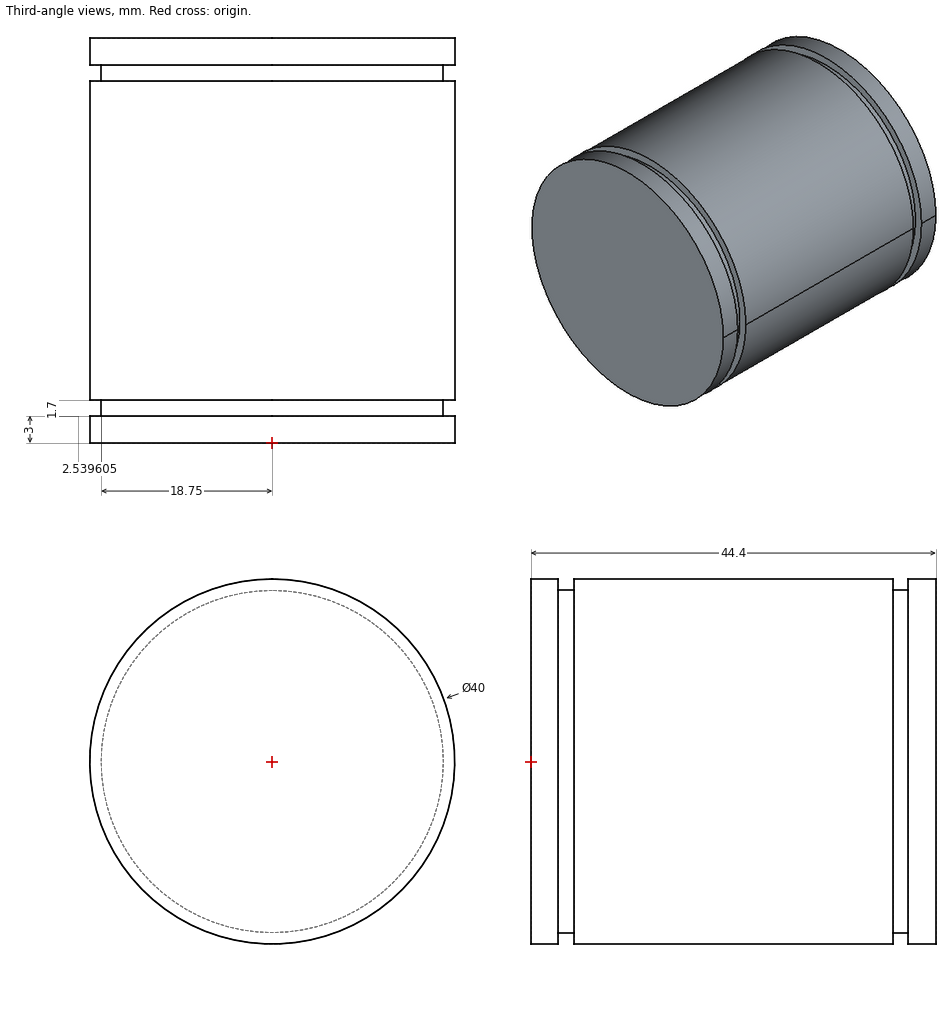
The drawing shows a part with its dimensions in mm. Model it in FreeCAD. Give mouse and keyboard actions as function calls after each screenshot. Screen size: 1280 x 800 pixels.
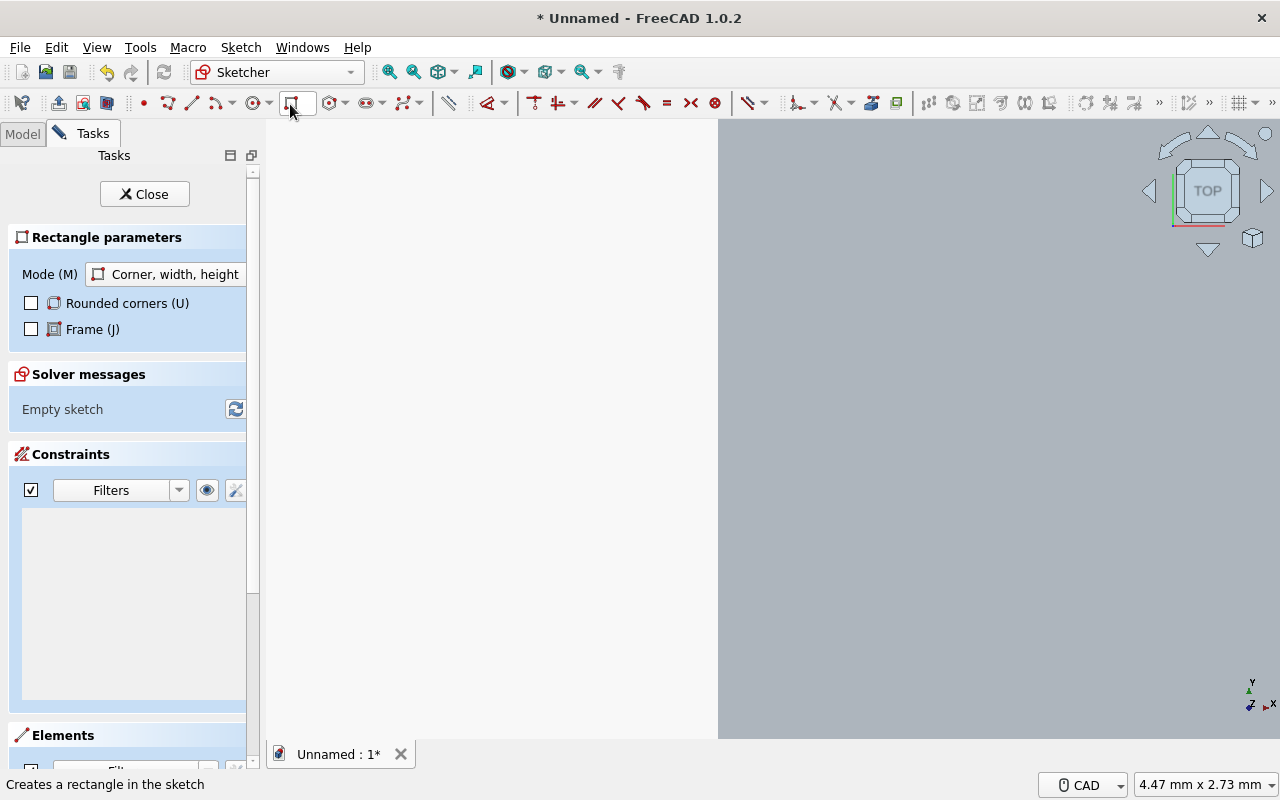
click(416, 236)
move(992, 622)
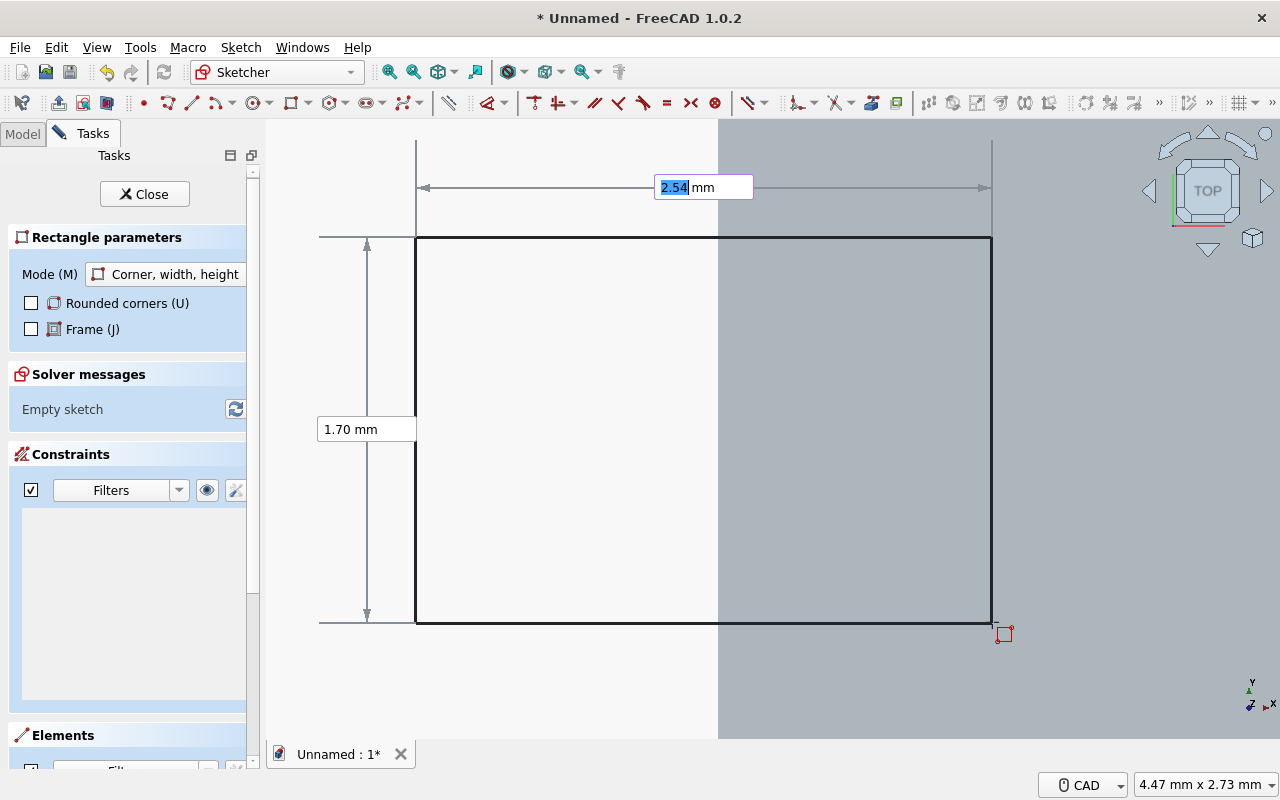
text(2.539605)
key(Tab)
text(1.7)
key(Return)
key(Escape)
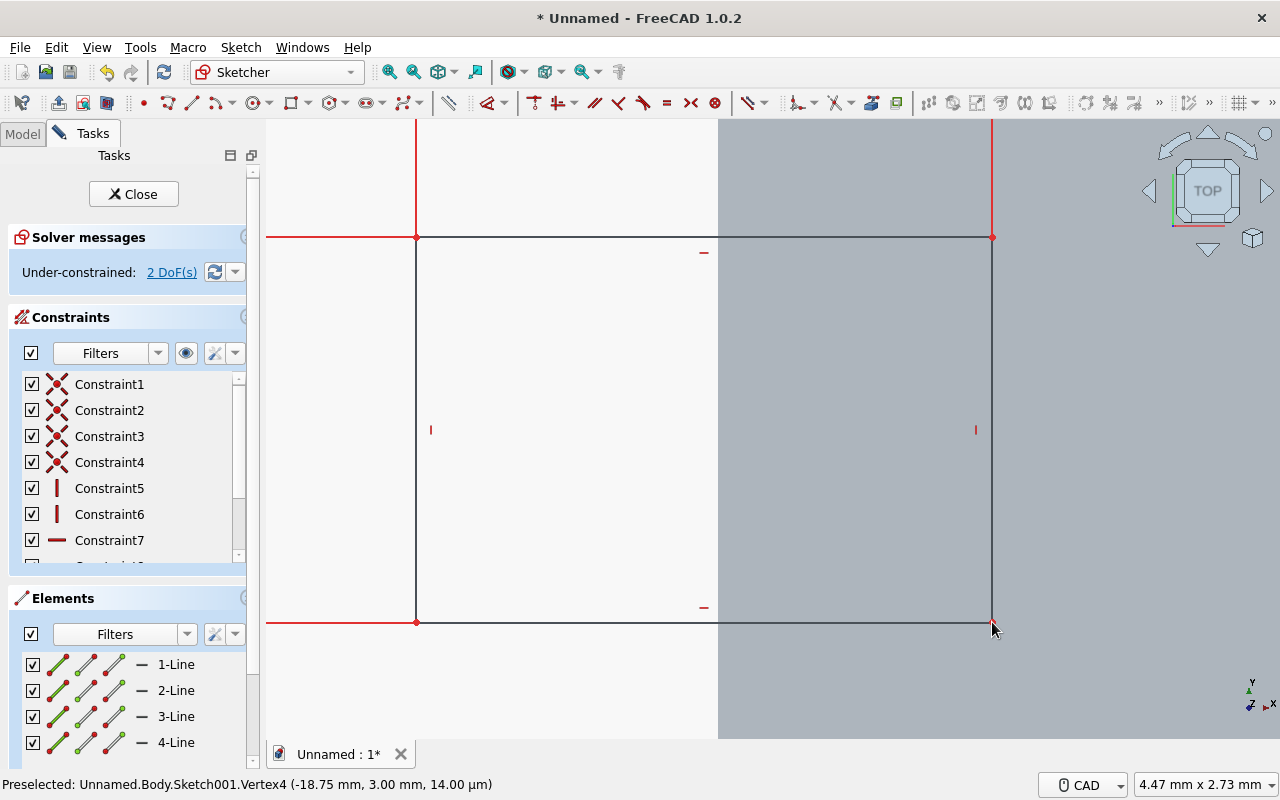
key(d)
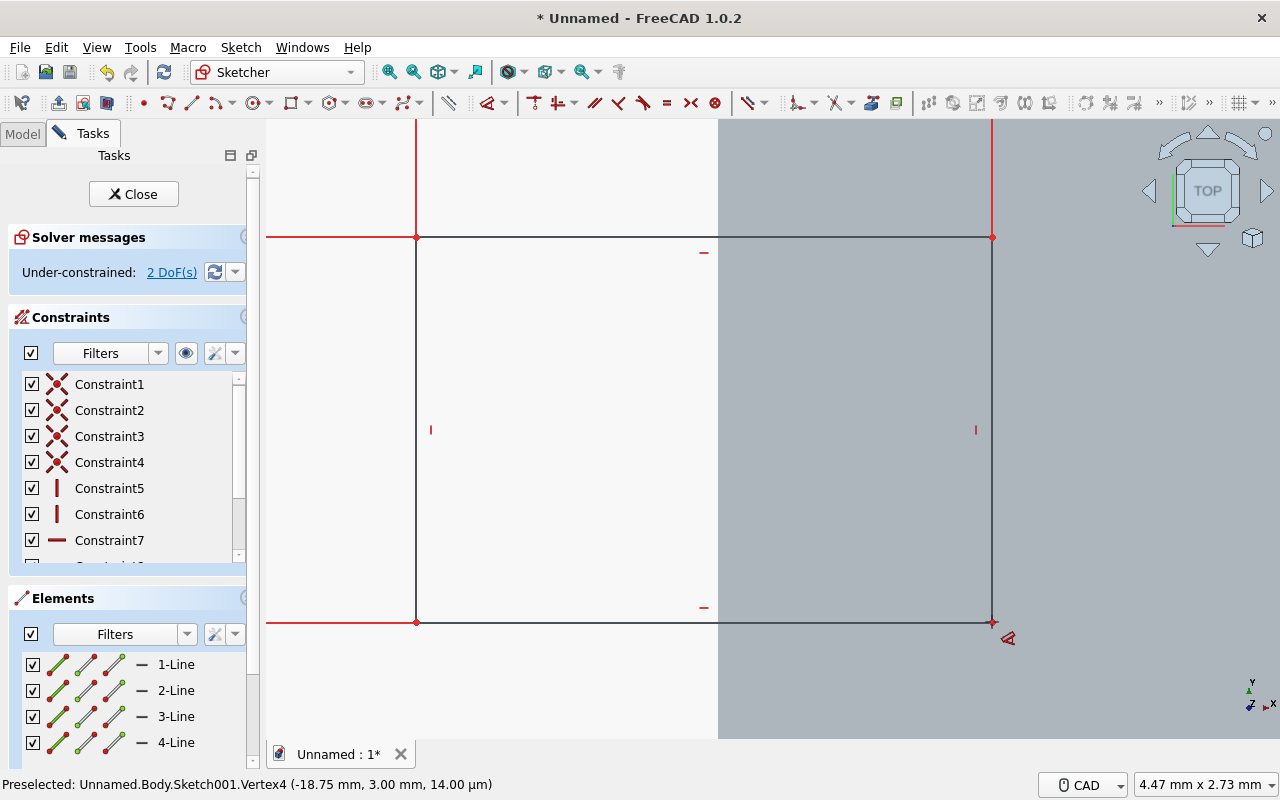
click(416, 623)
click(382, 667)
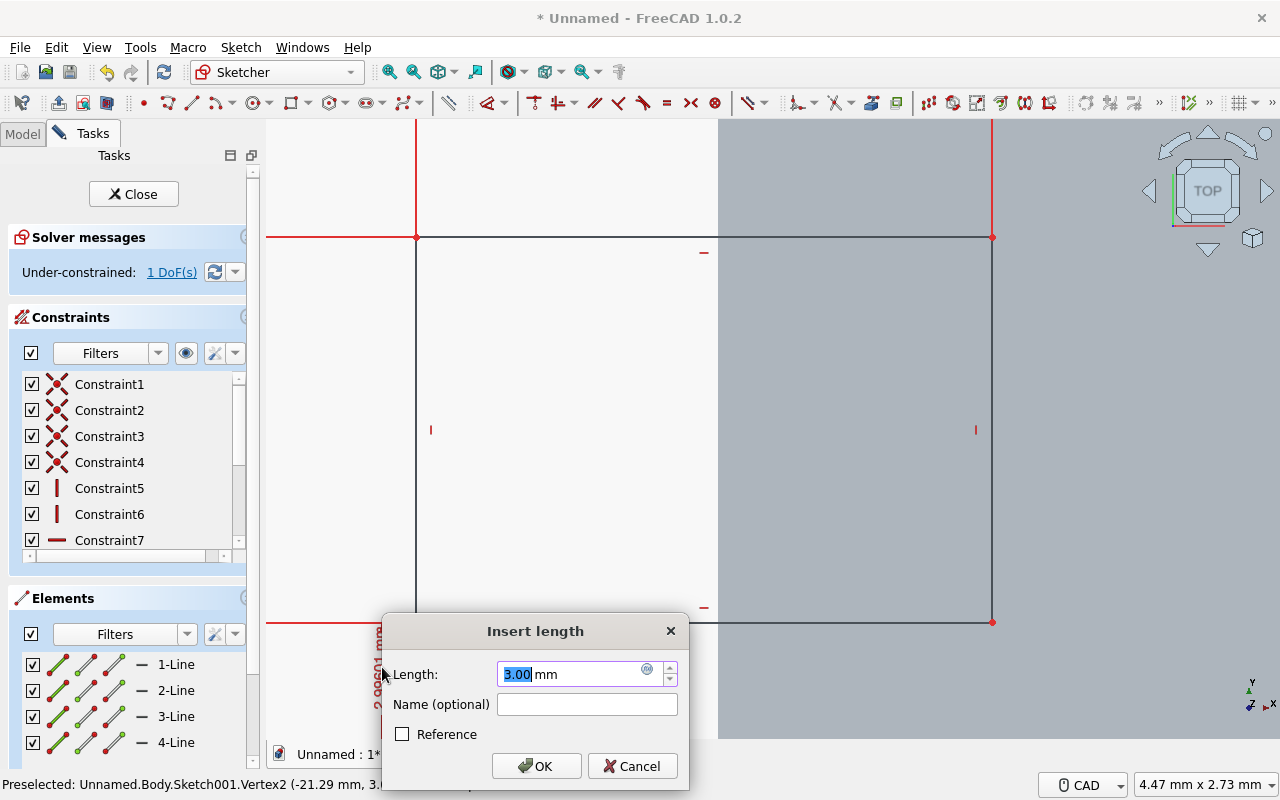
text(3)
key(Return)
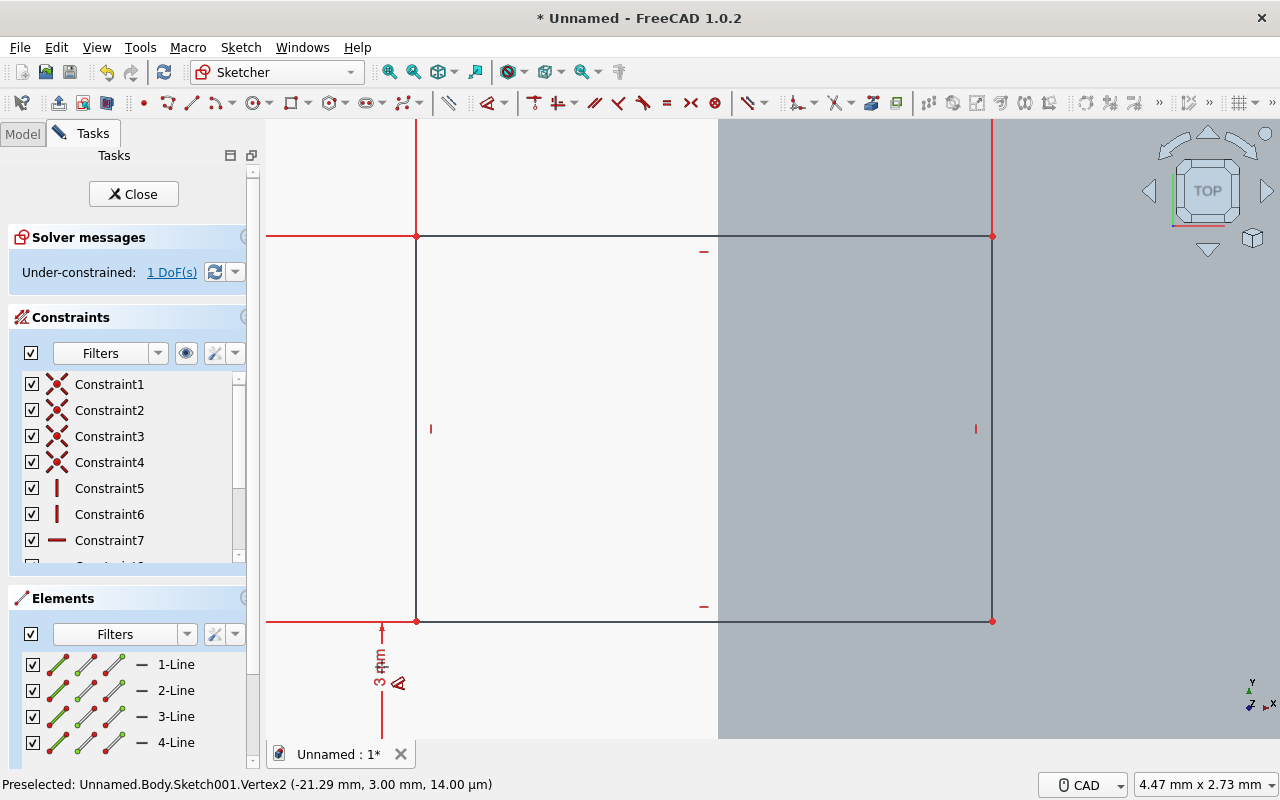
click(992, 622)
click(1054, 588)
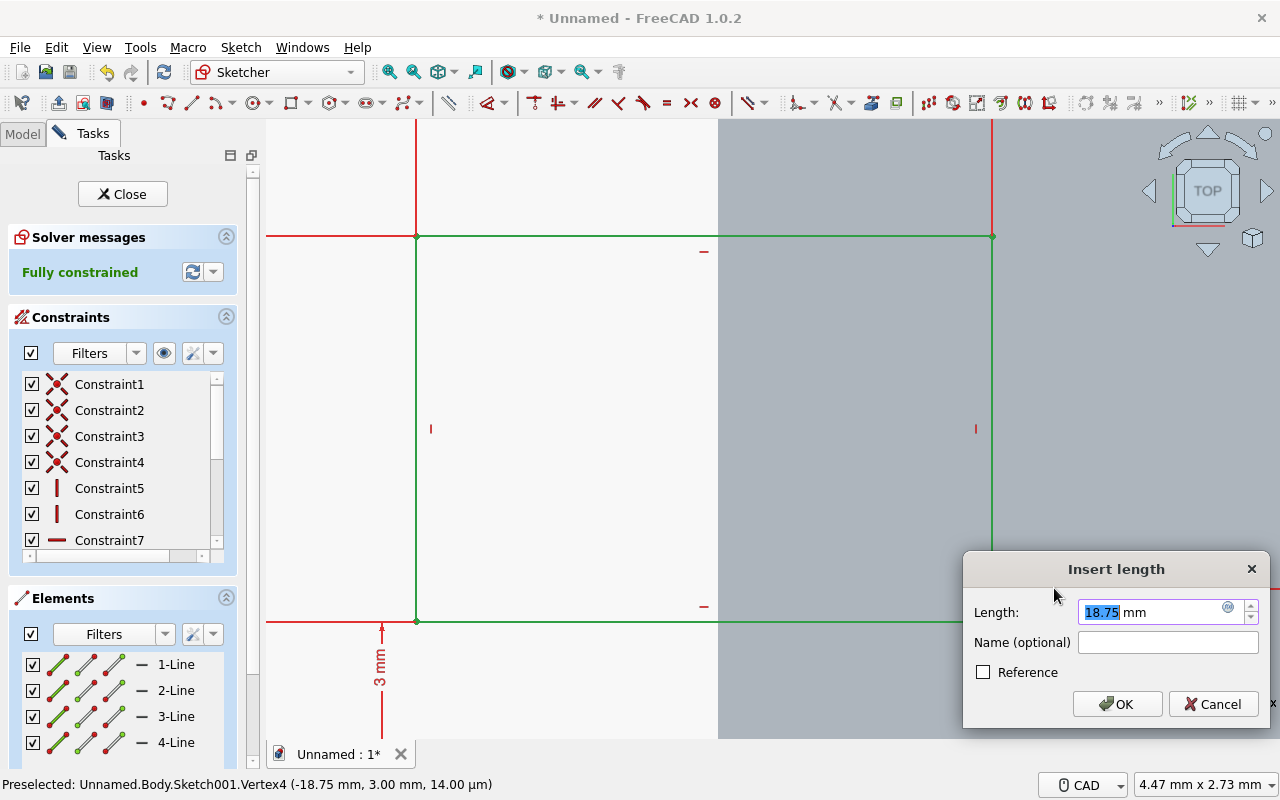
text(18.75)
key(Return)
key(Escape)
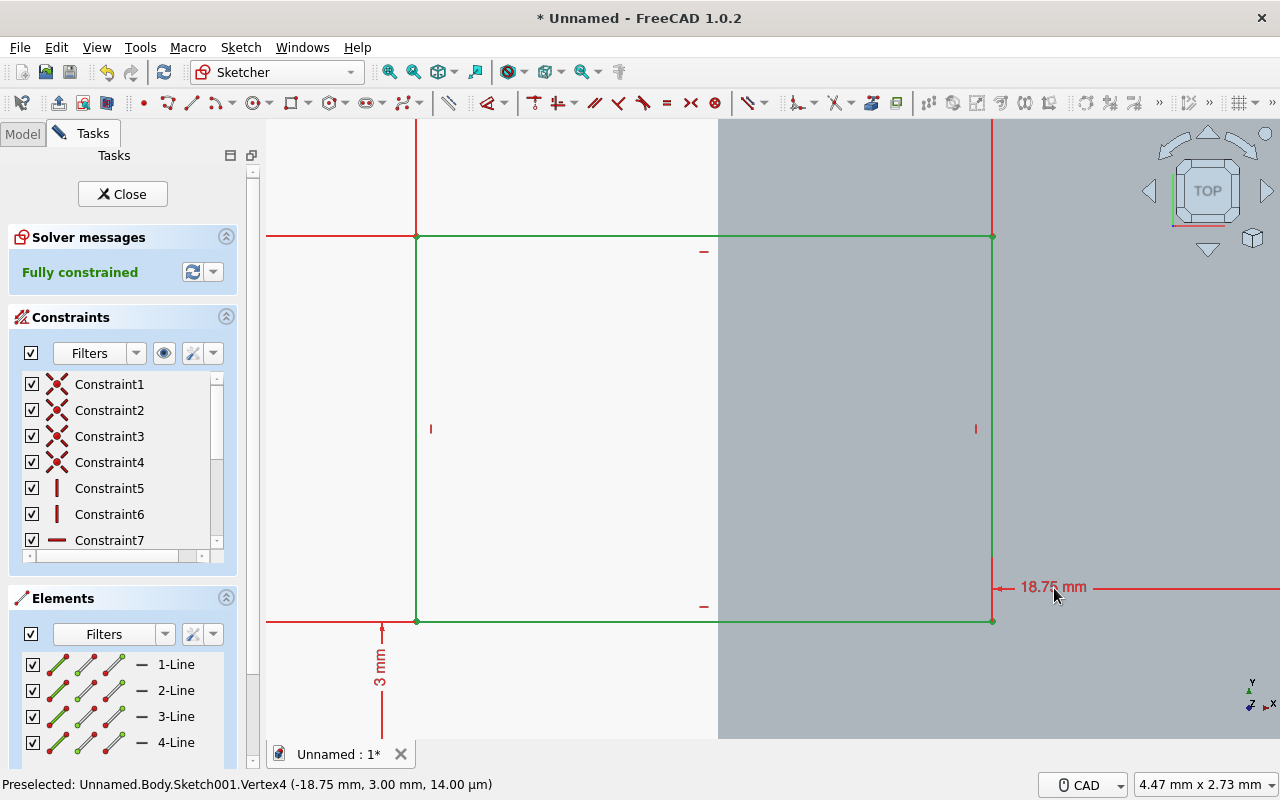
click(123, 194)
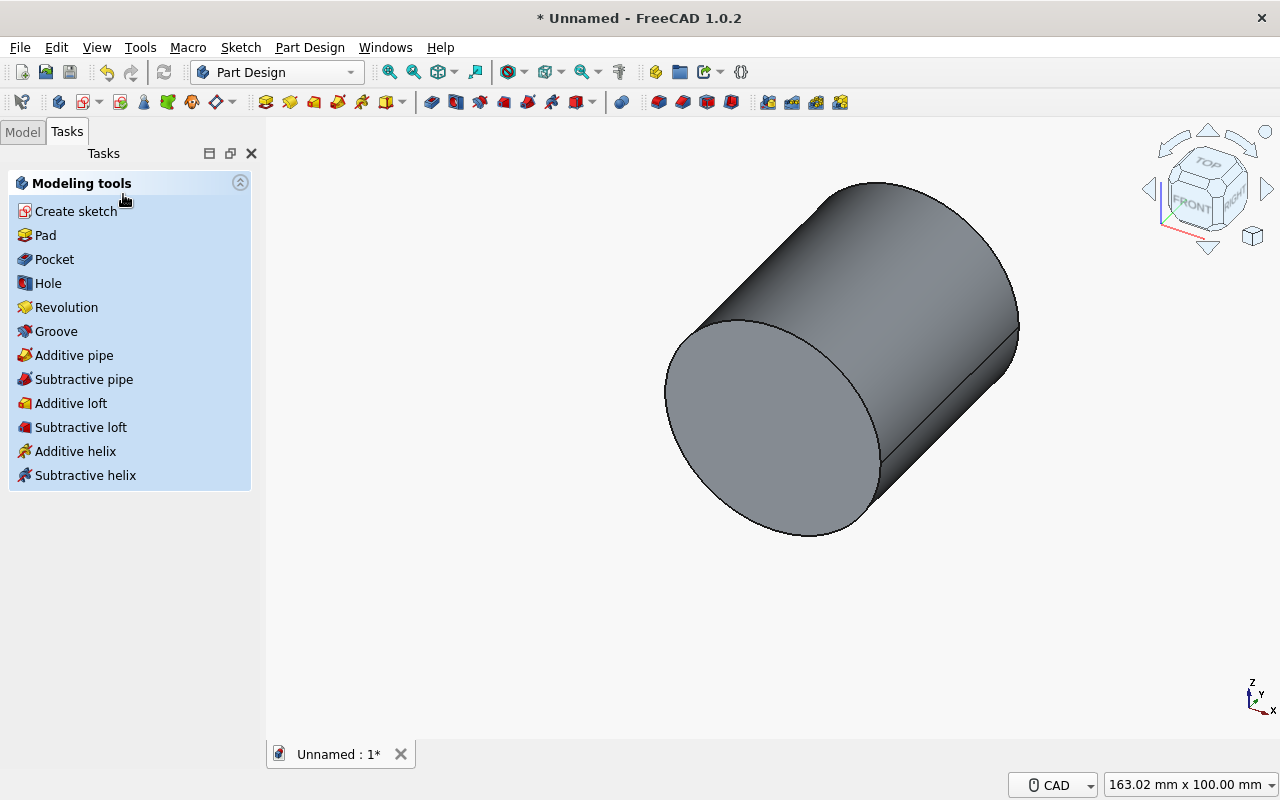
click(480, 102)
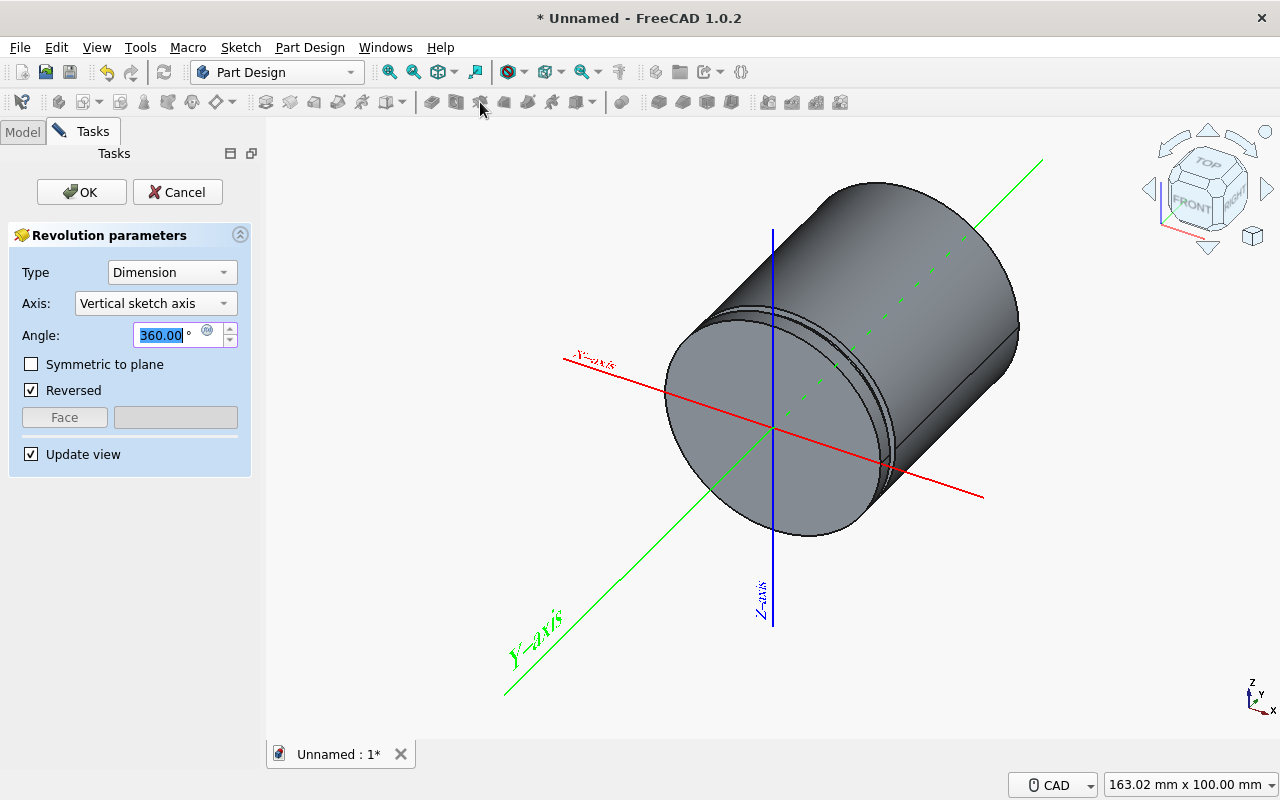
click(82, 192)